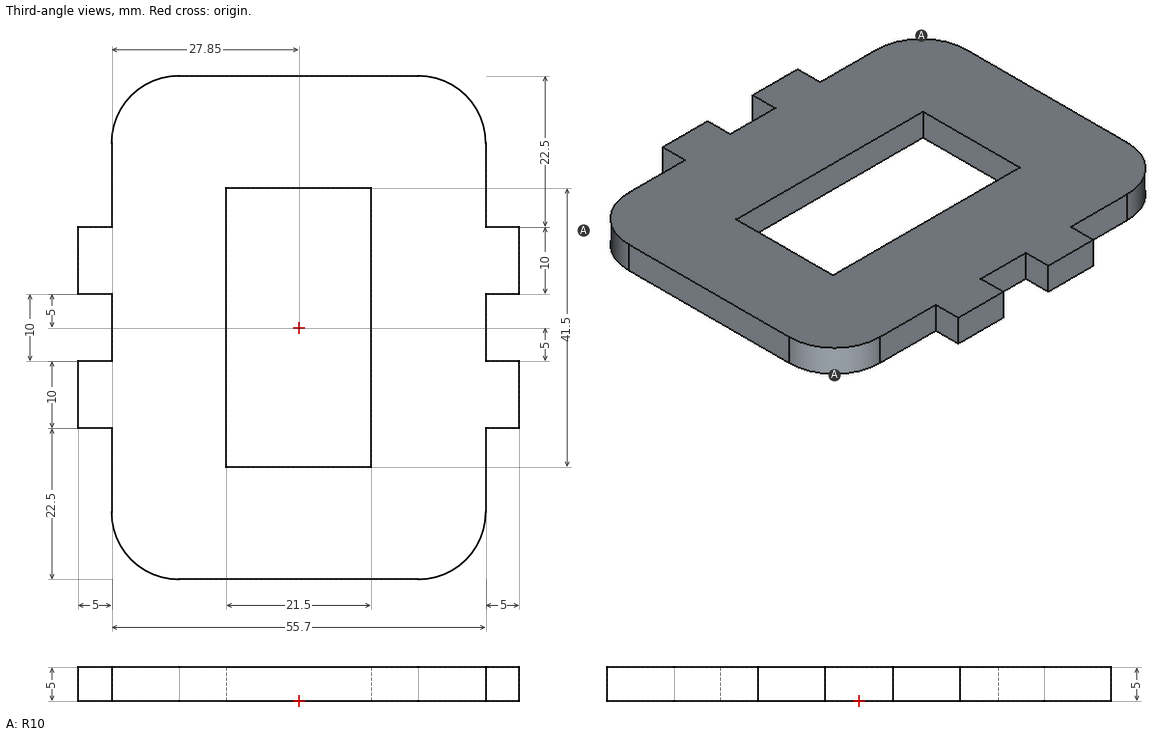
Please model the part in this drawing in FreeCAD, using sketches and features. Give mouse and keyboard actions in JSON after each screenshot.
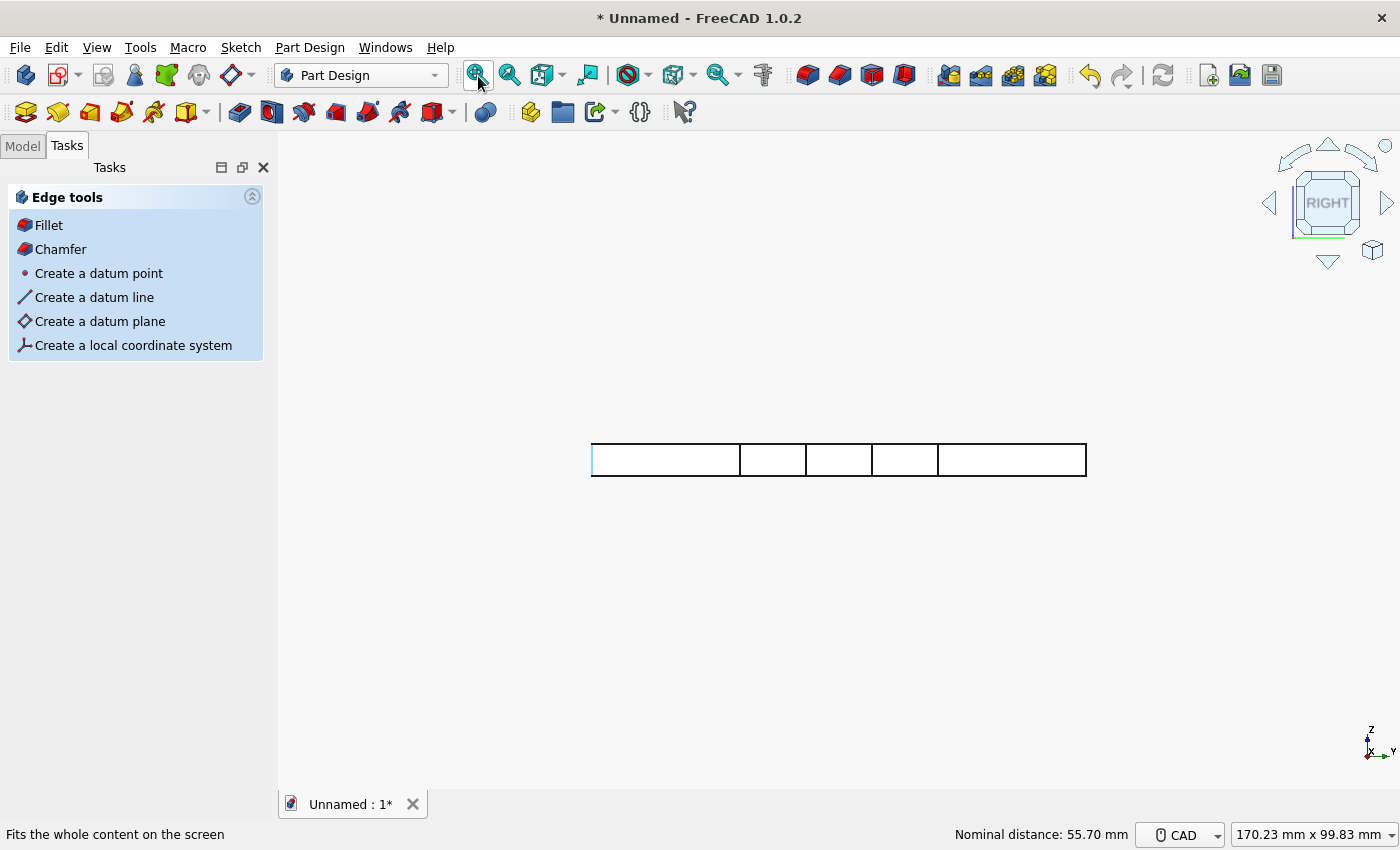
{"action": "left_click", "coordinate": [1086, 459], "text": "ctrl"}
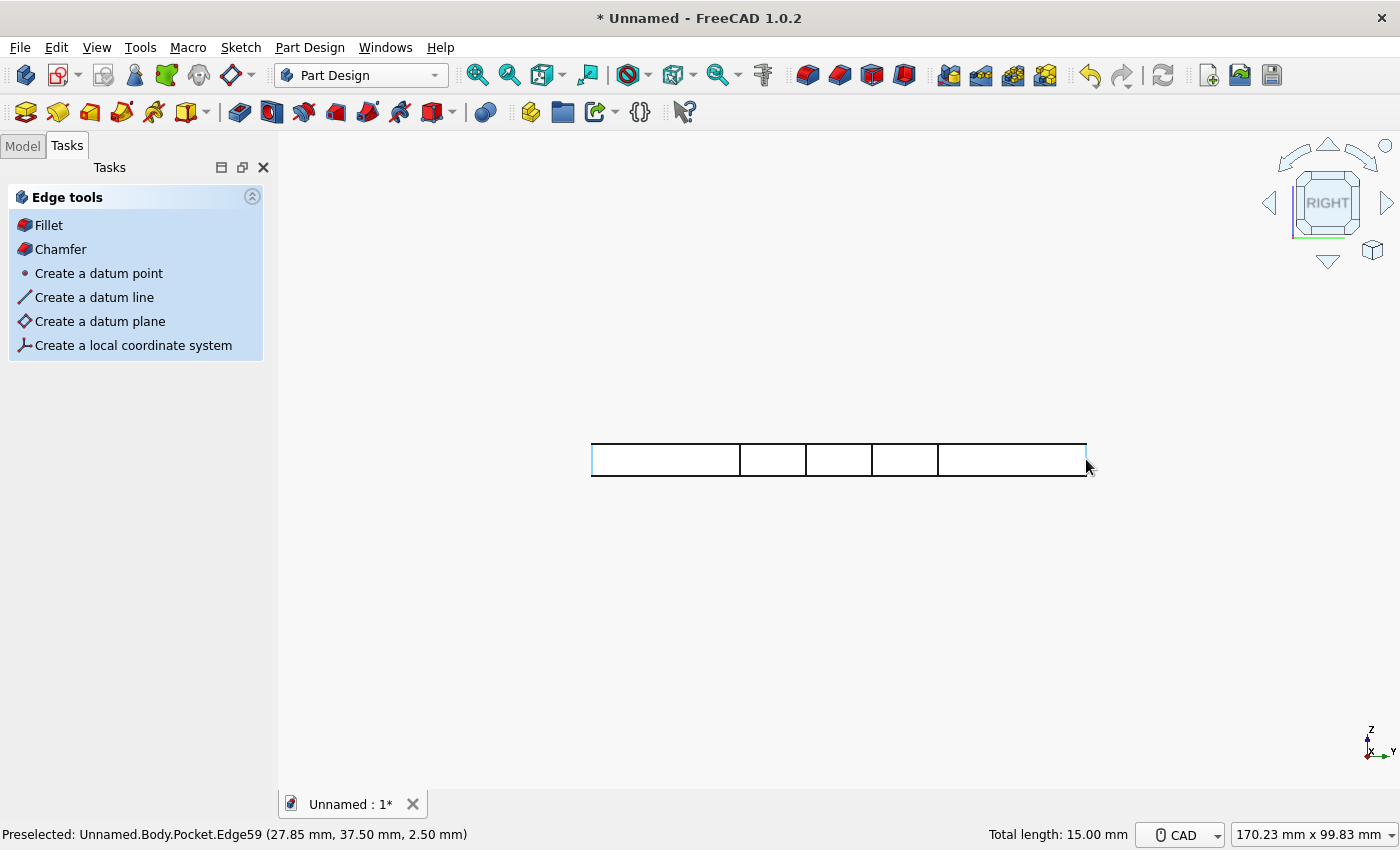
{"action": "key", "text": "5"}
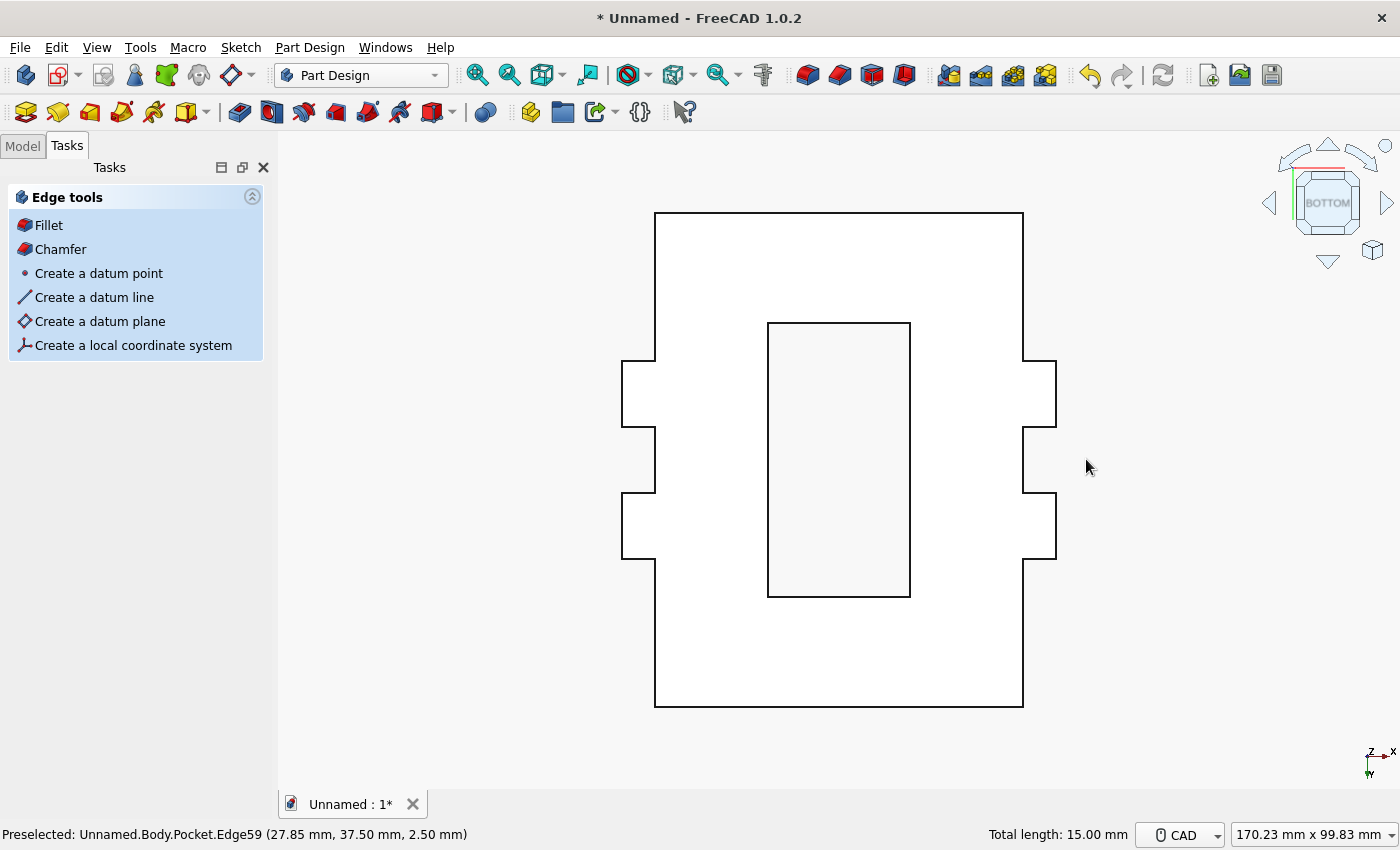
{"action": "key", "text": "4"}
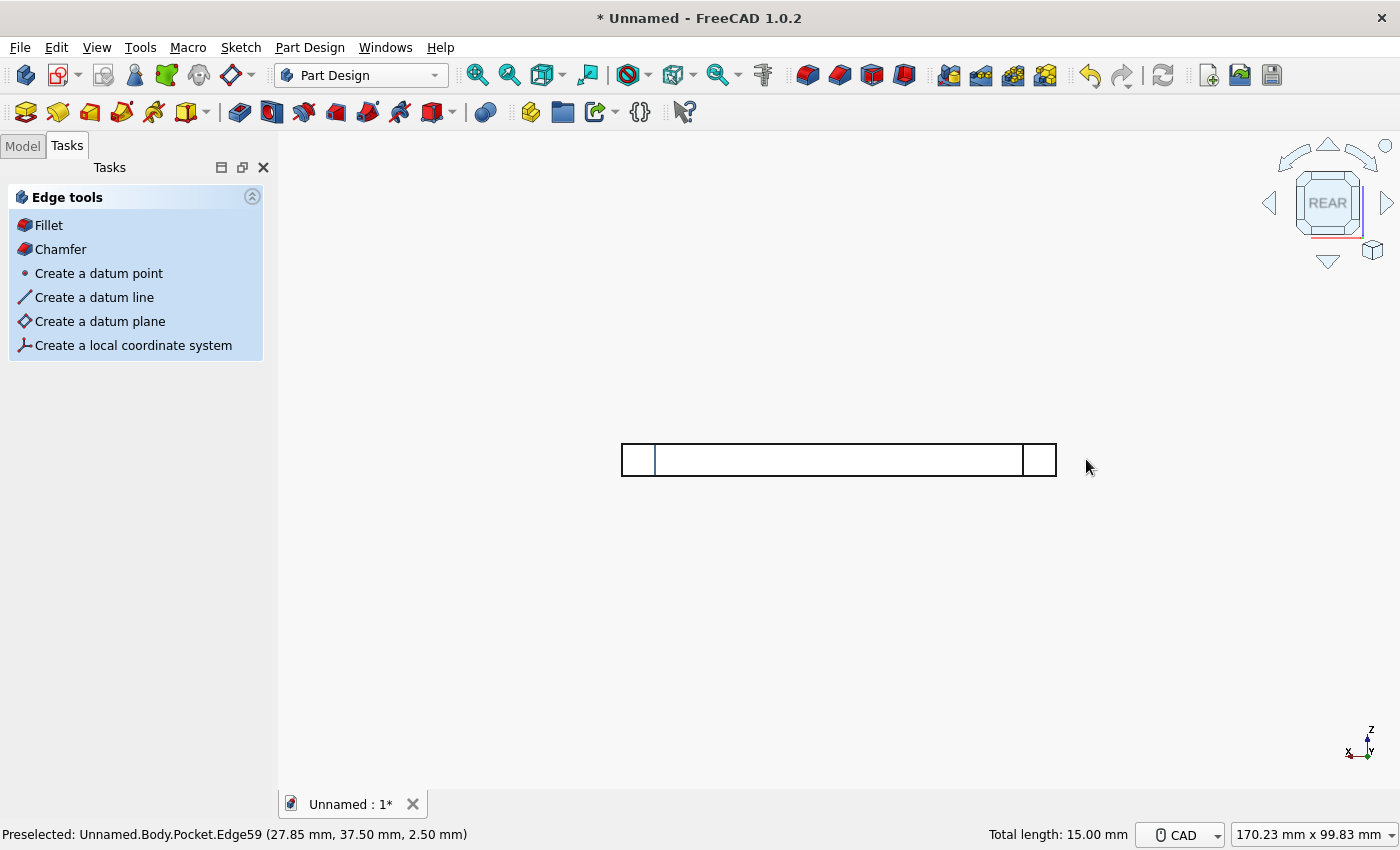
{"action": "key", "text": "v f"}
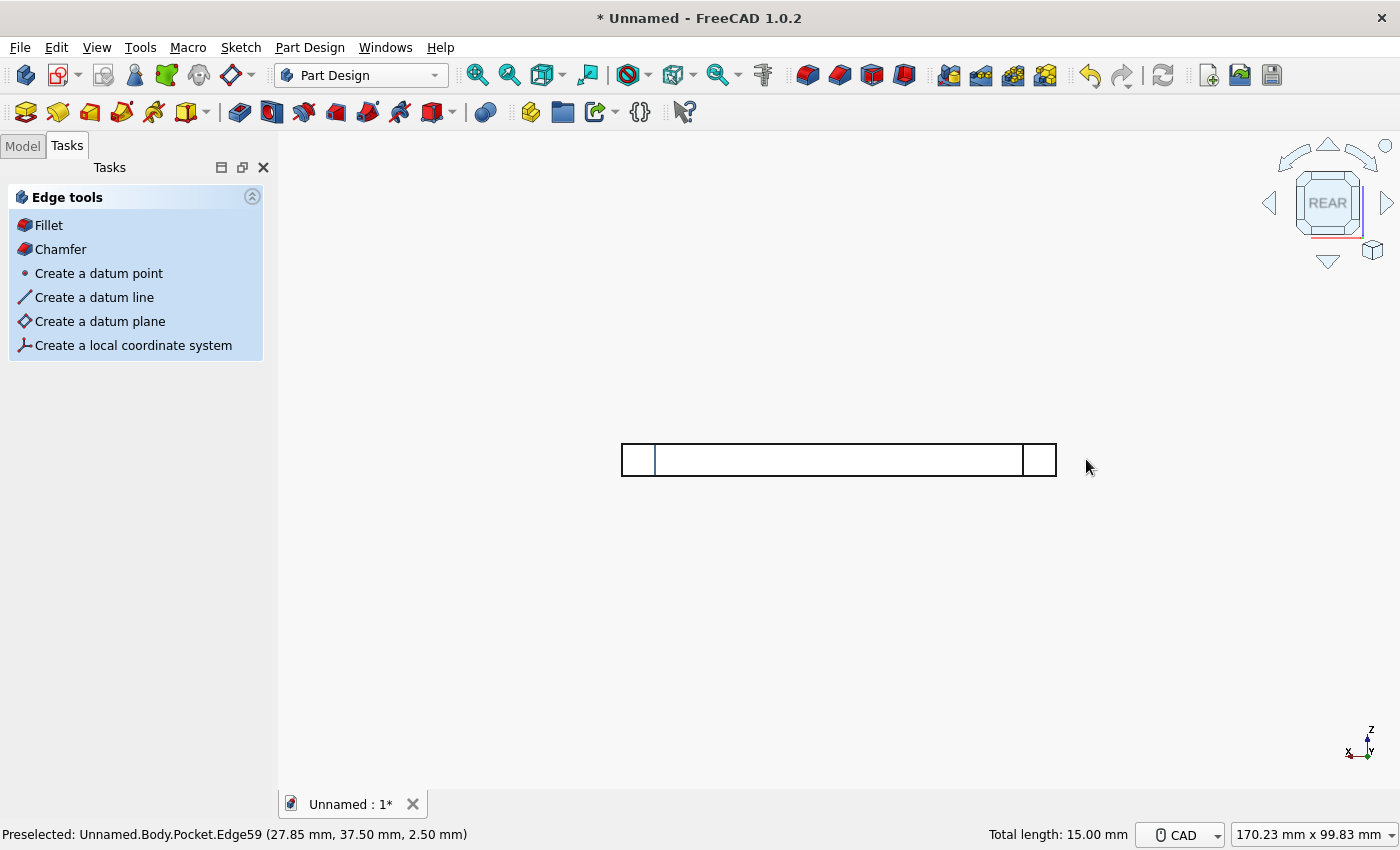
{"action": "left_click", "coordinate": [1023, 459], "text": "ctrl"}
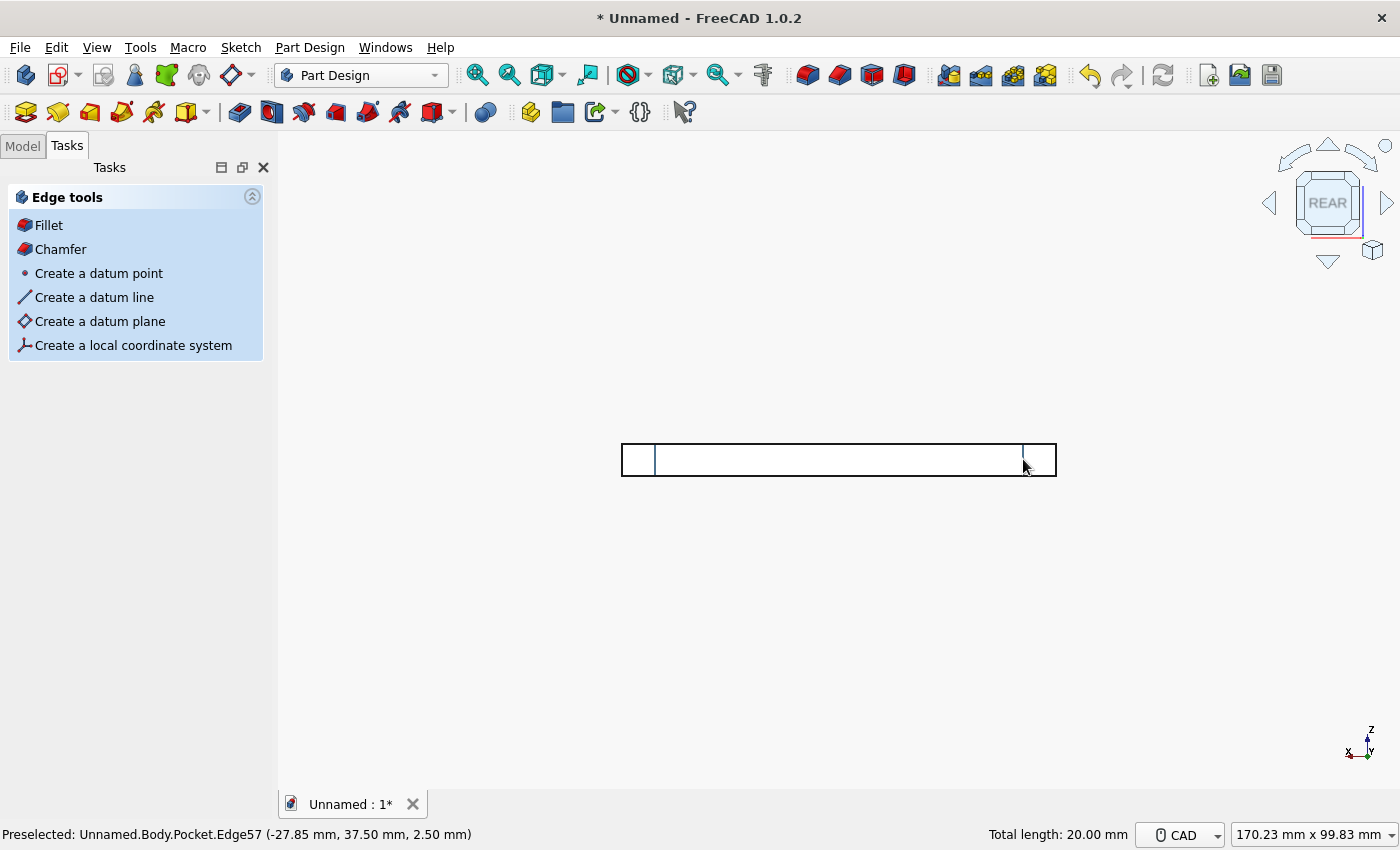
{"action": "left_click", "coordinate": [808, 76]}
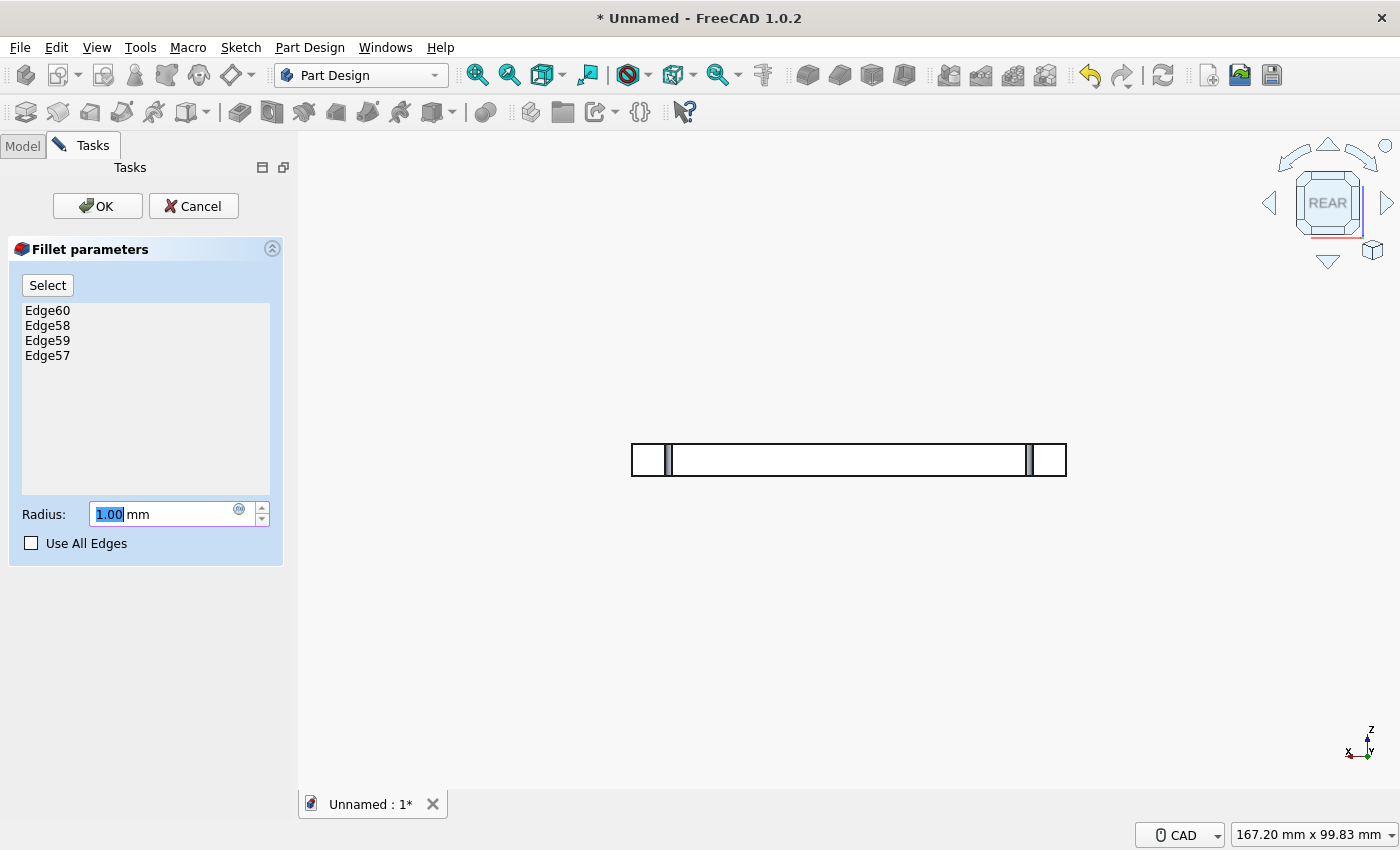
{"action": "type", "text": "10"}
{"action": "key", "text": "Tab"}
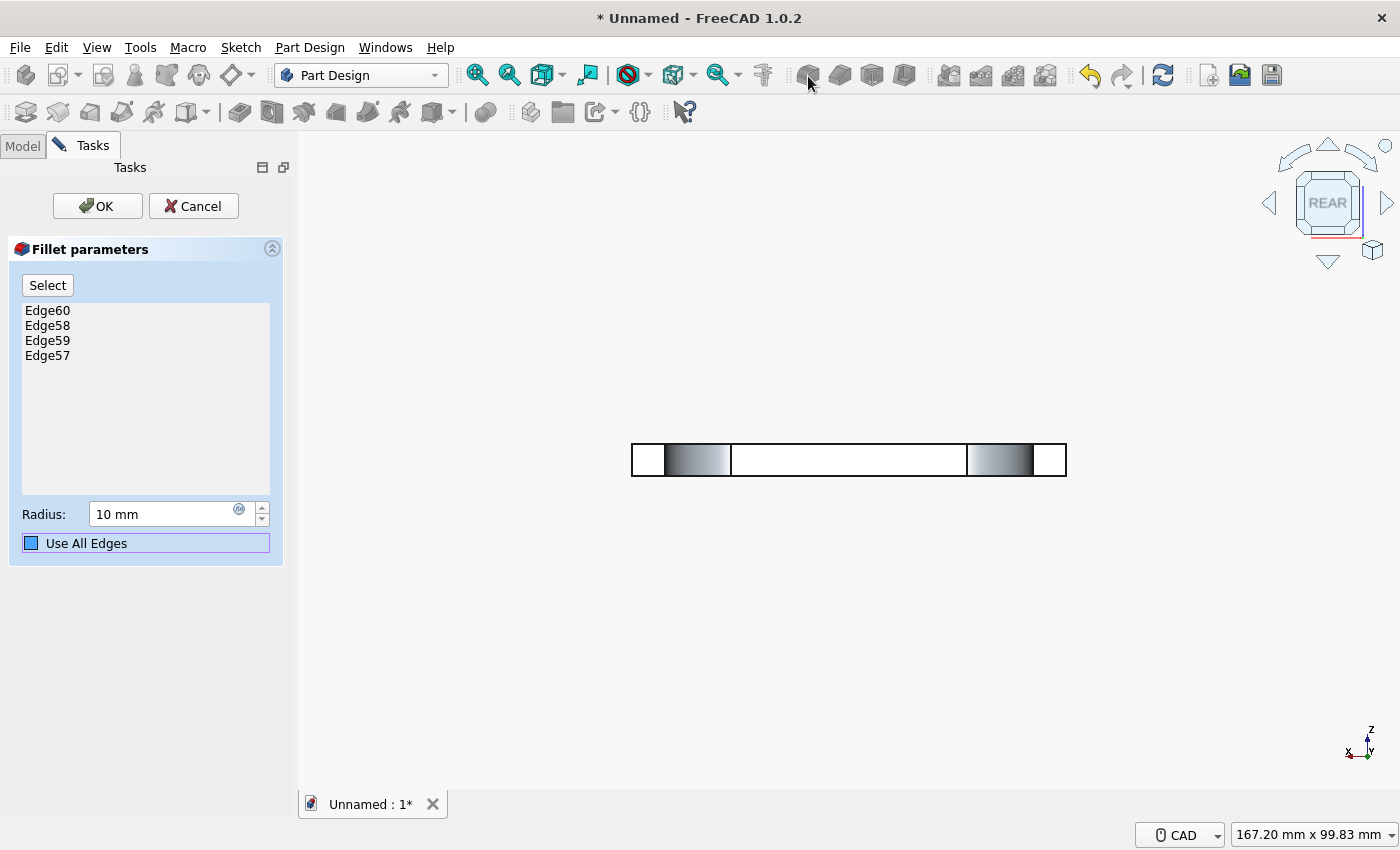
{"action": "left_click", "coordinate": [98, 206]}